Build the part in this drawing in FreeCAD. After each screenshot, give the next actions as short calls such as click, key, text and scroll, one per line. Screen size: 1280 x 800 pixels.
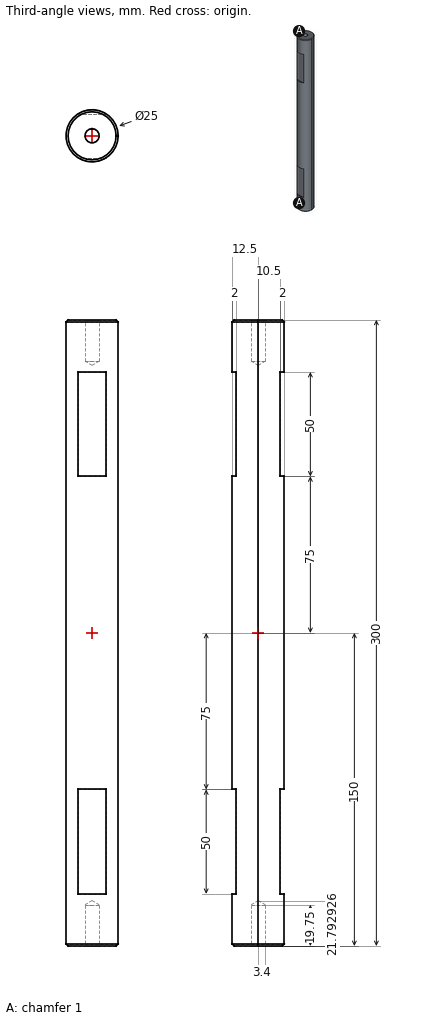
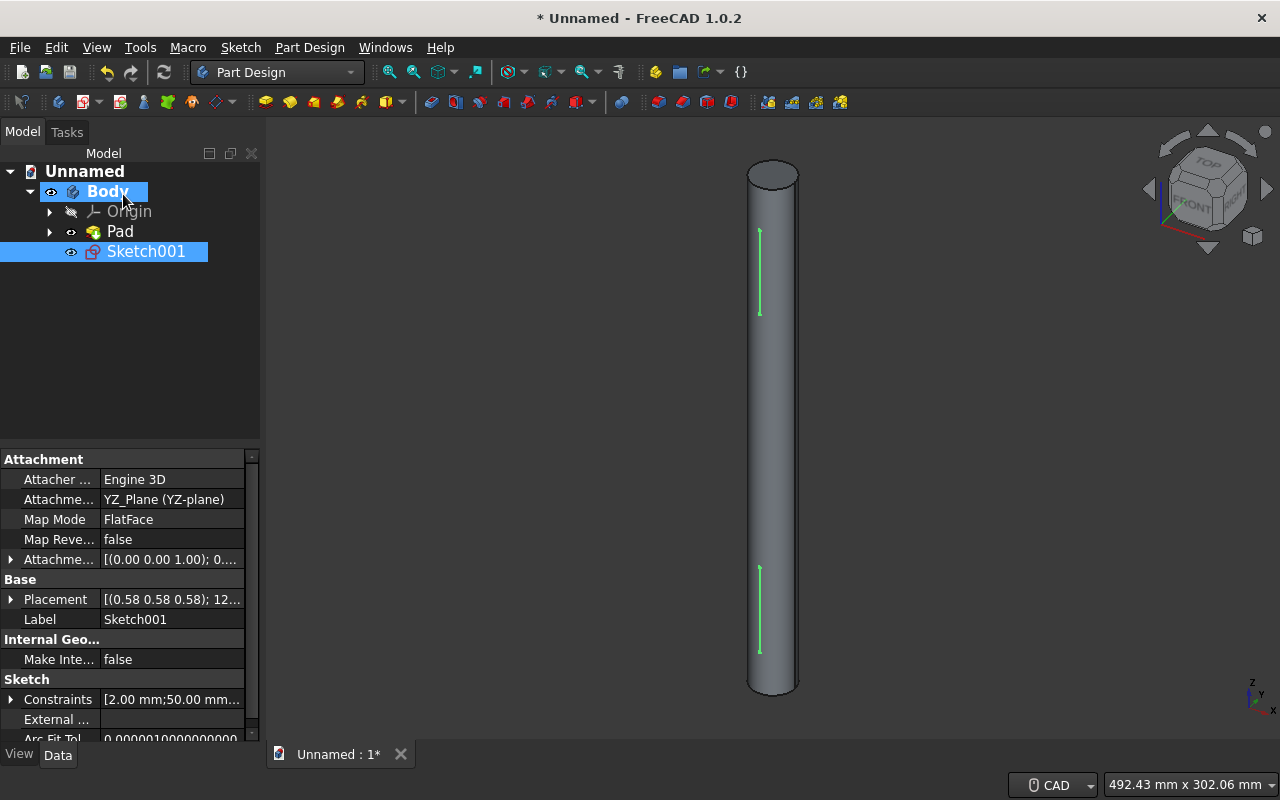
click(432, 102)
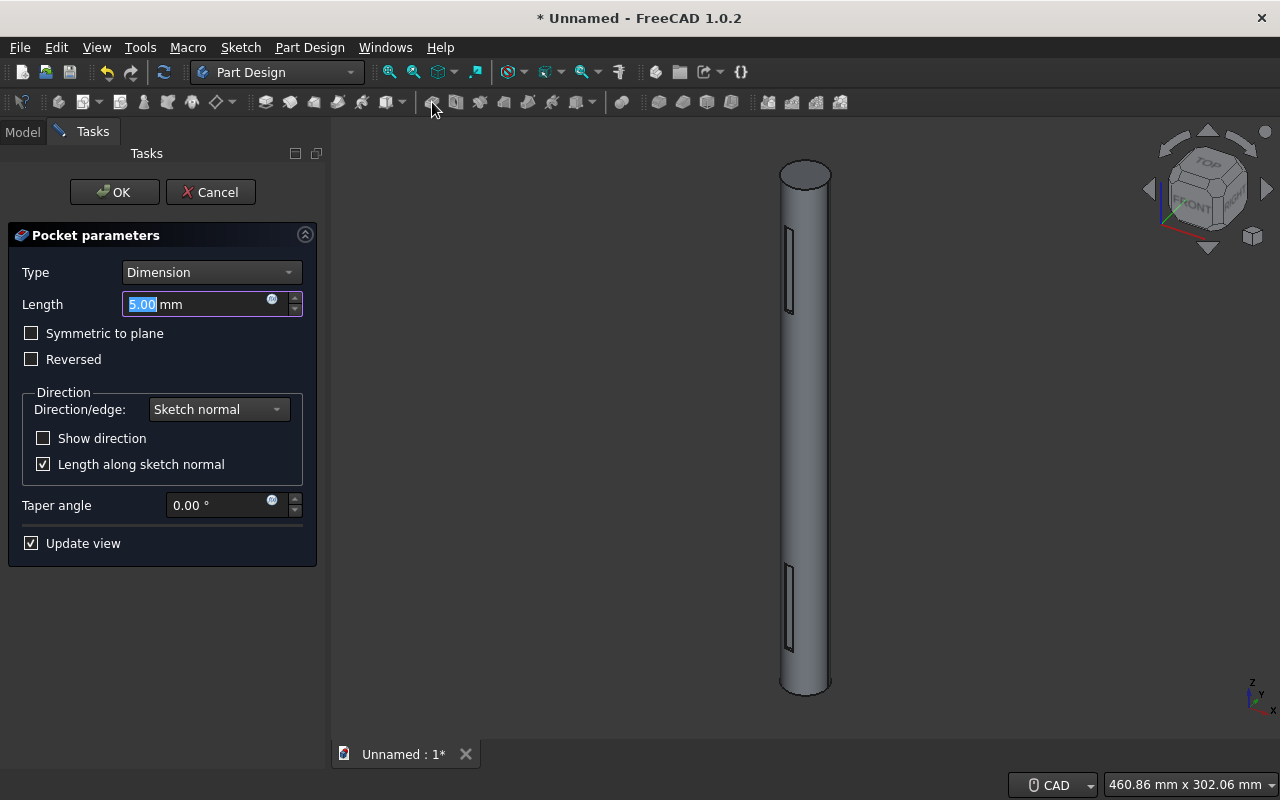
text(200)
key(Tab)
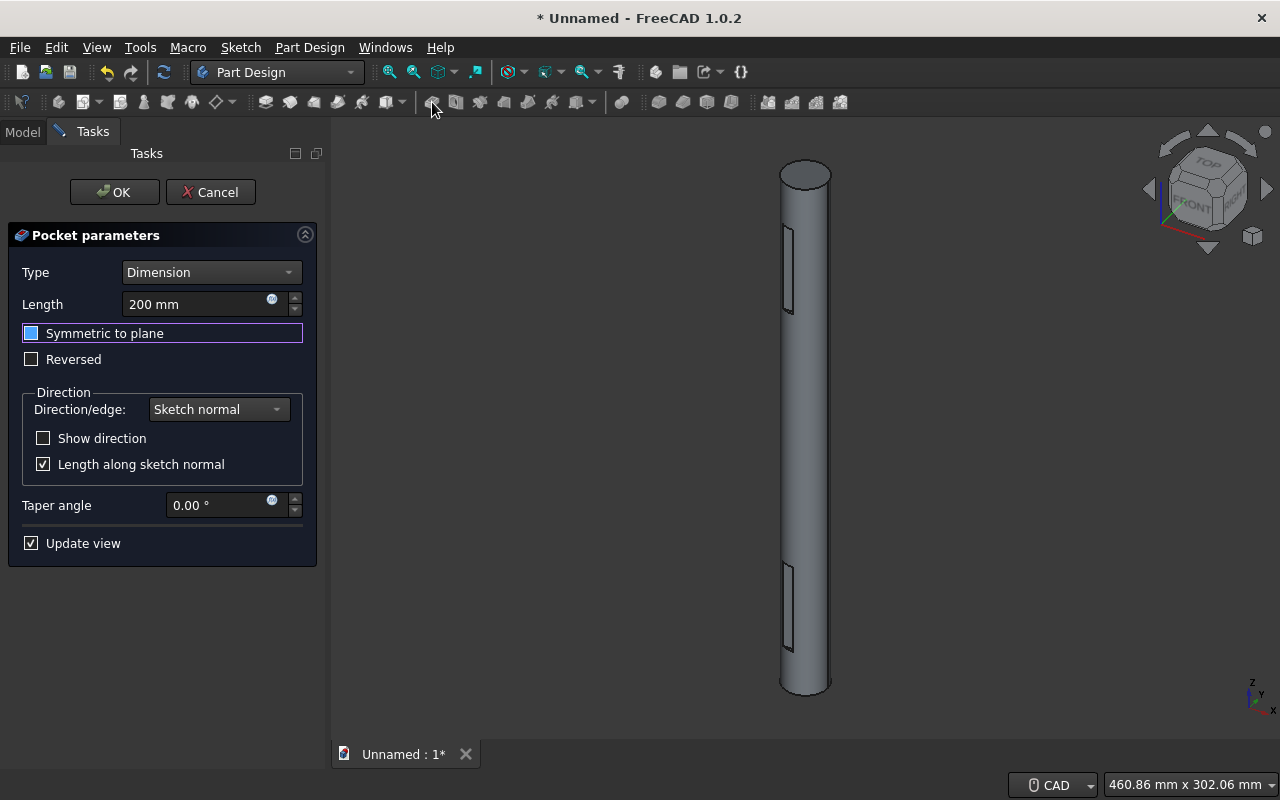
click(30, 333)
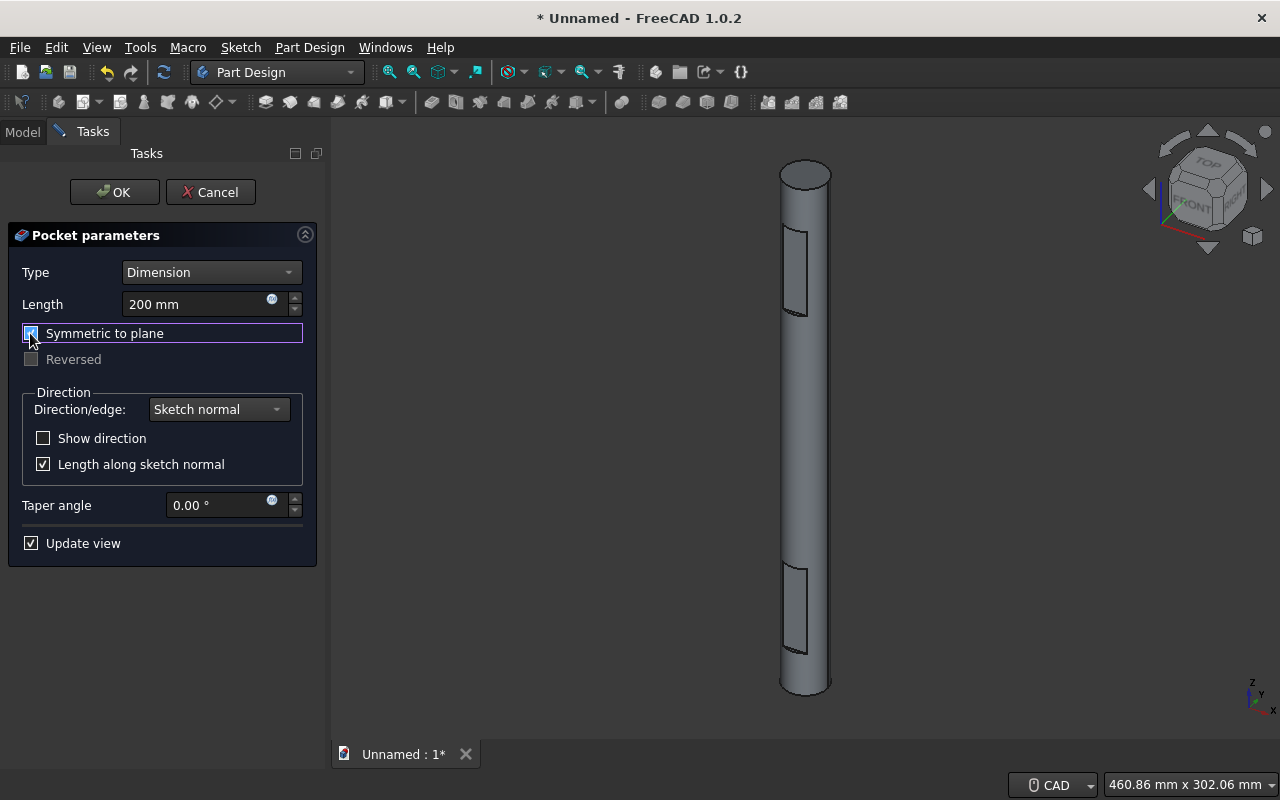
click(115, 192)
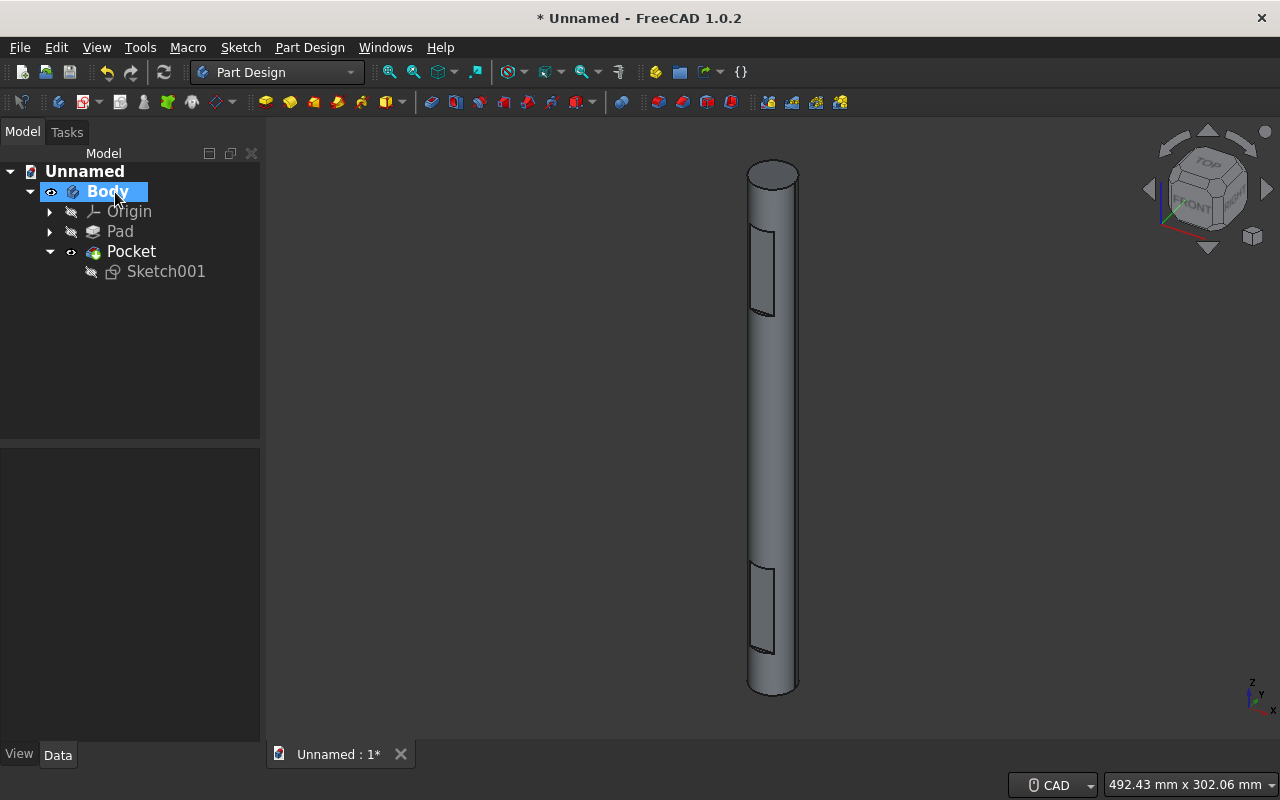
click(747, 176)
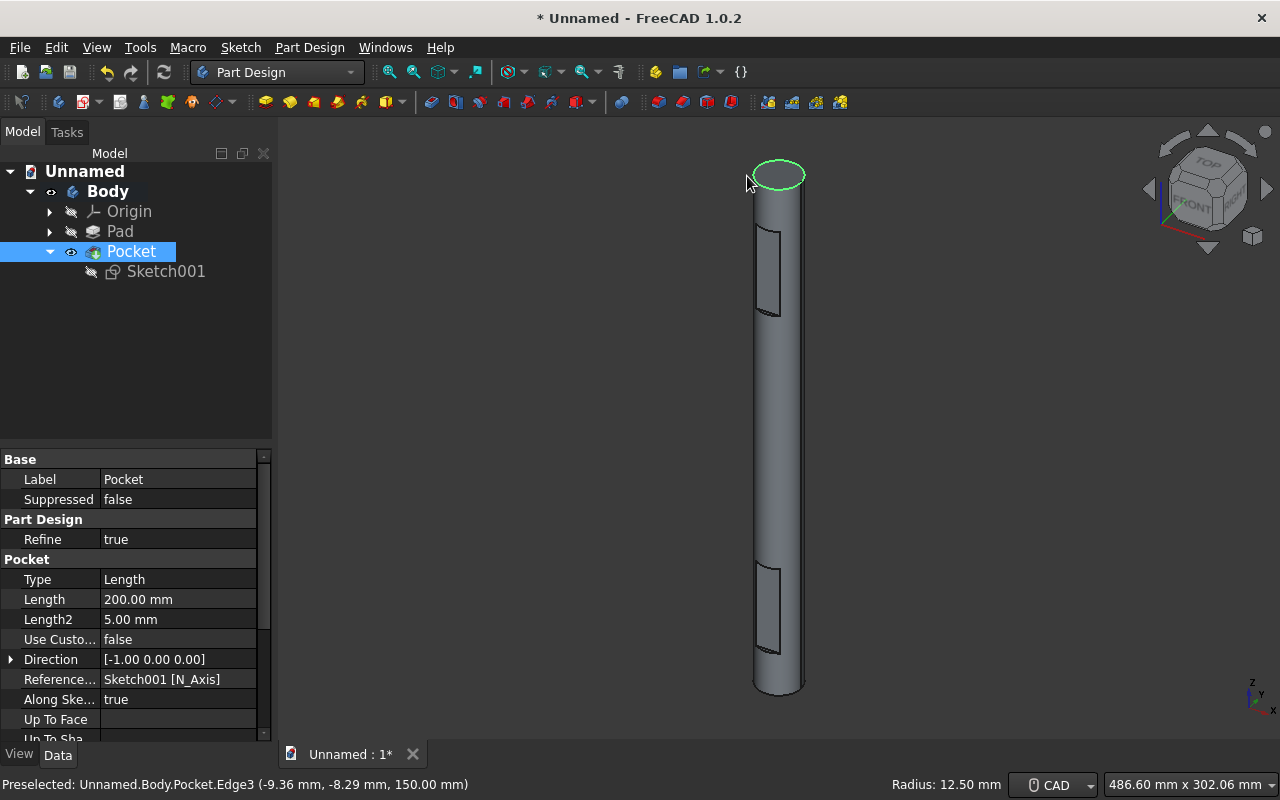
key(0)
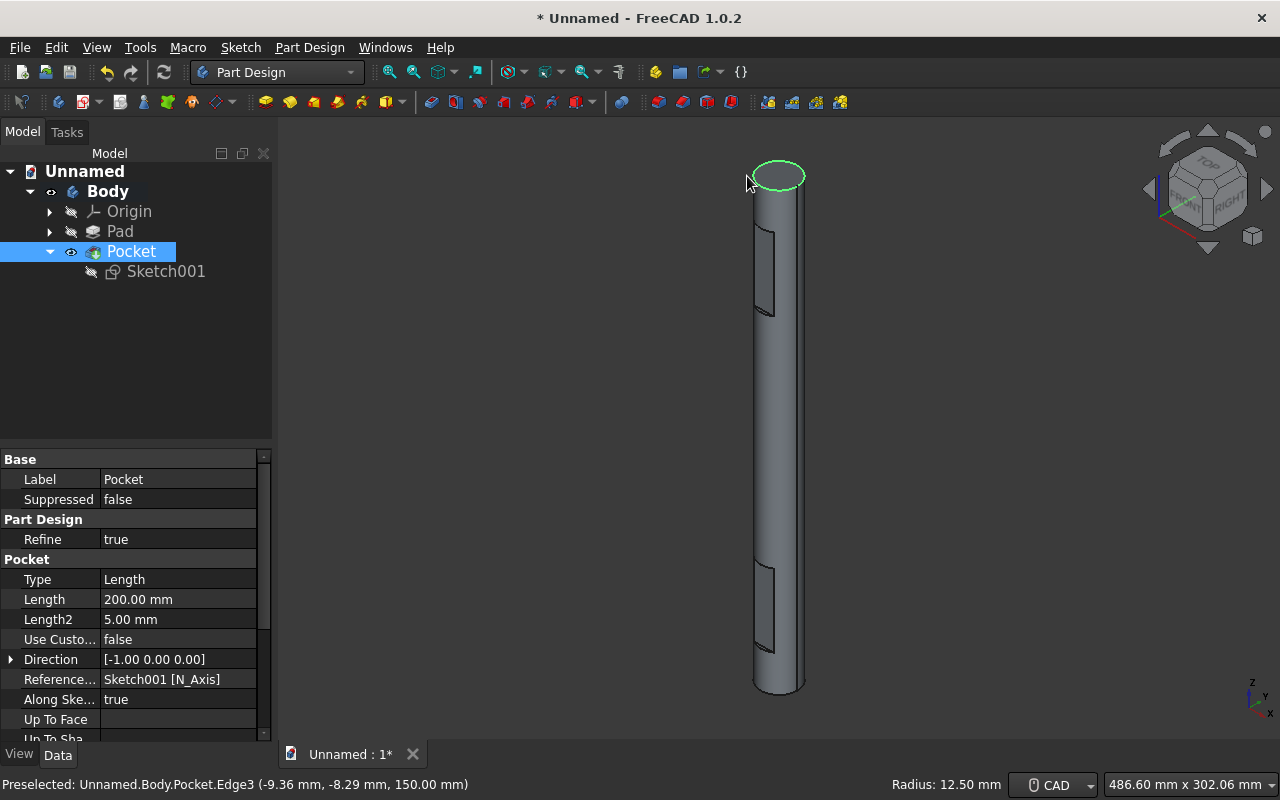
click(756, 686, ctrl)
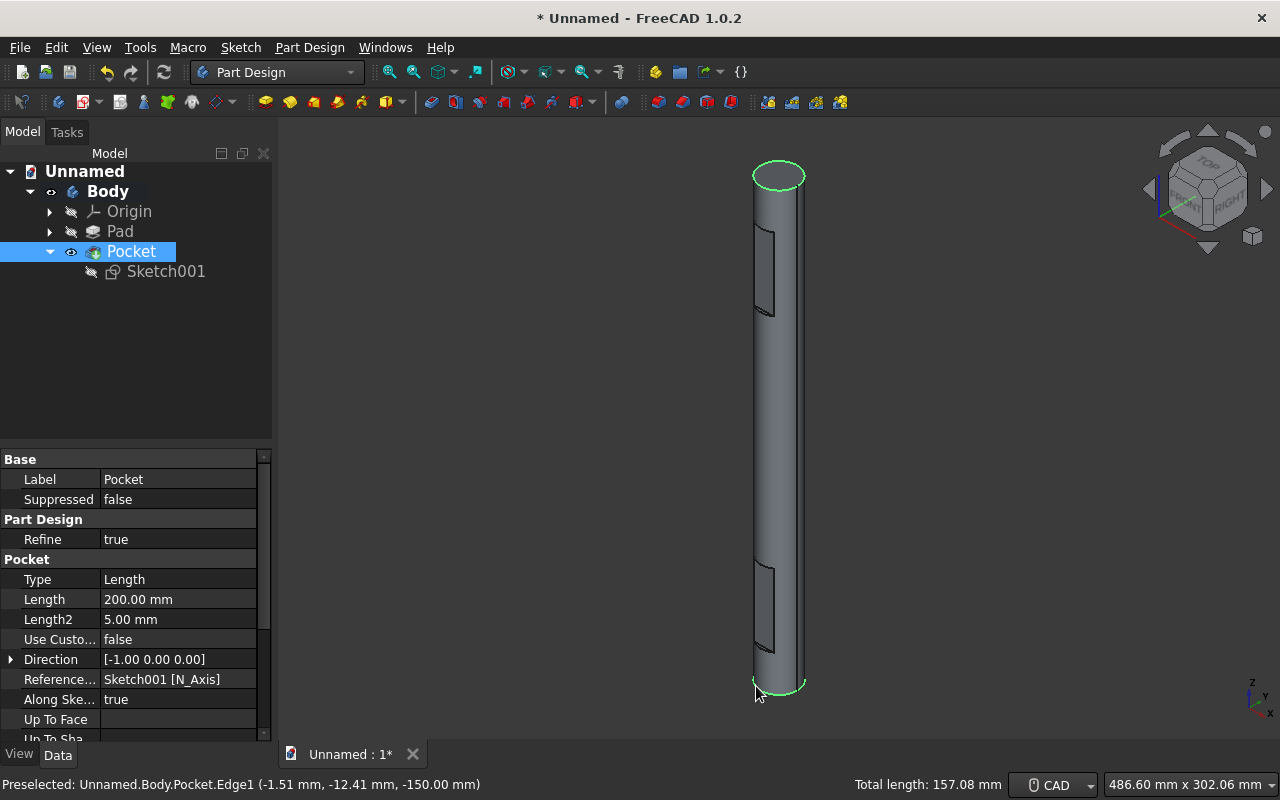
click(684, 102)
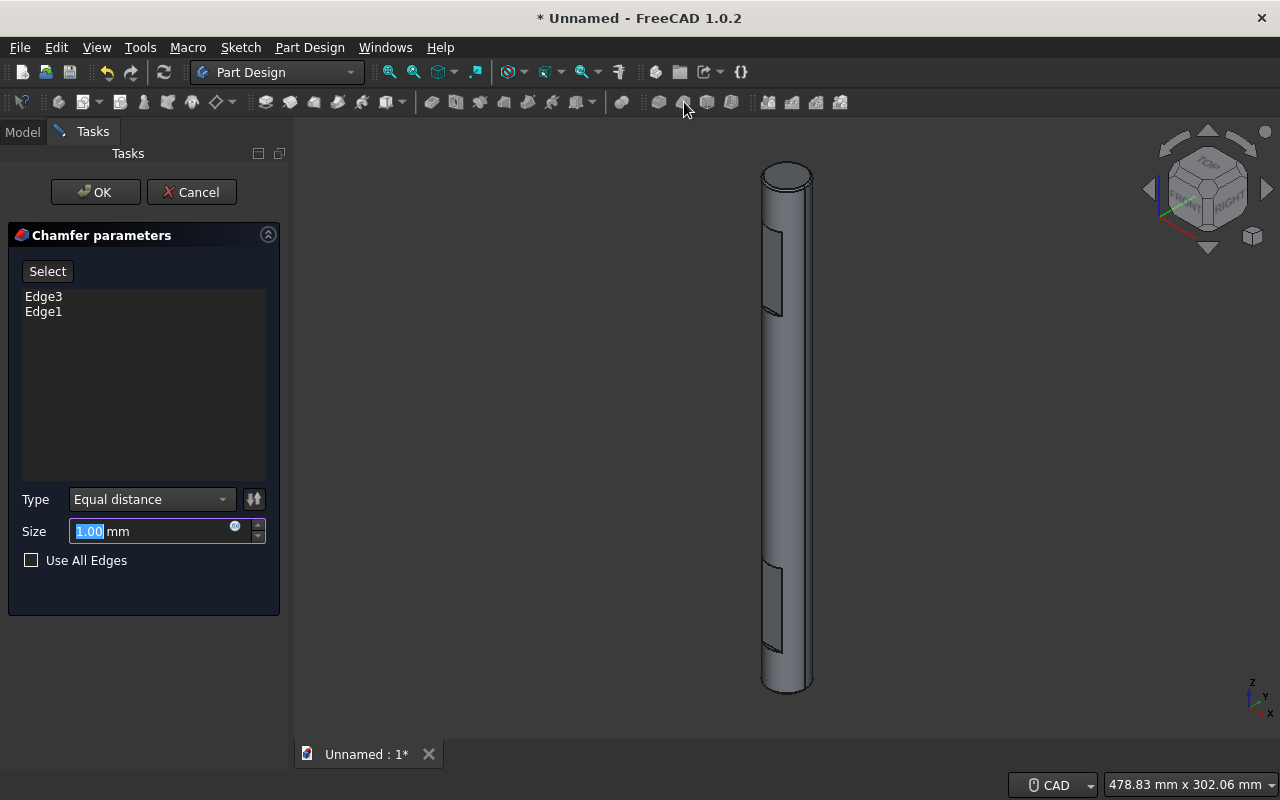
text(1)
key(Tab)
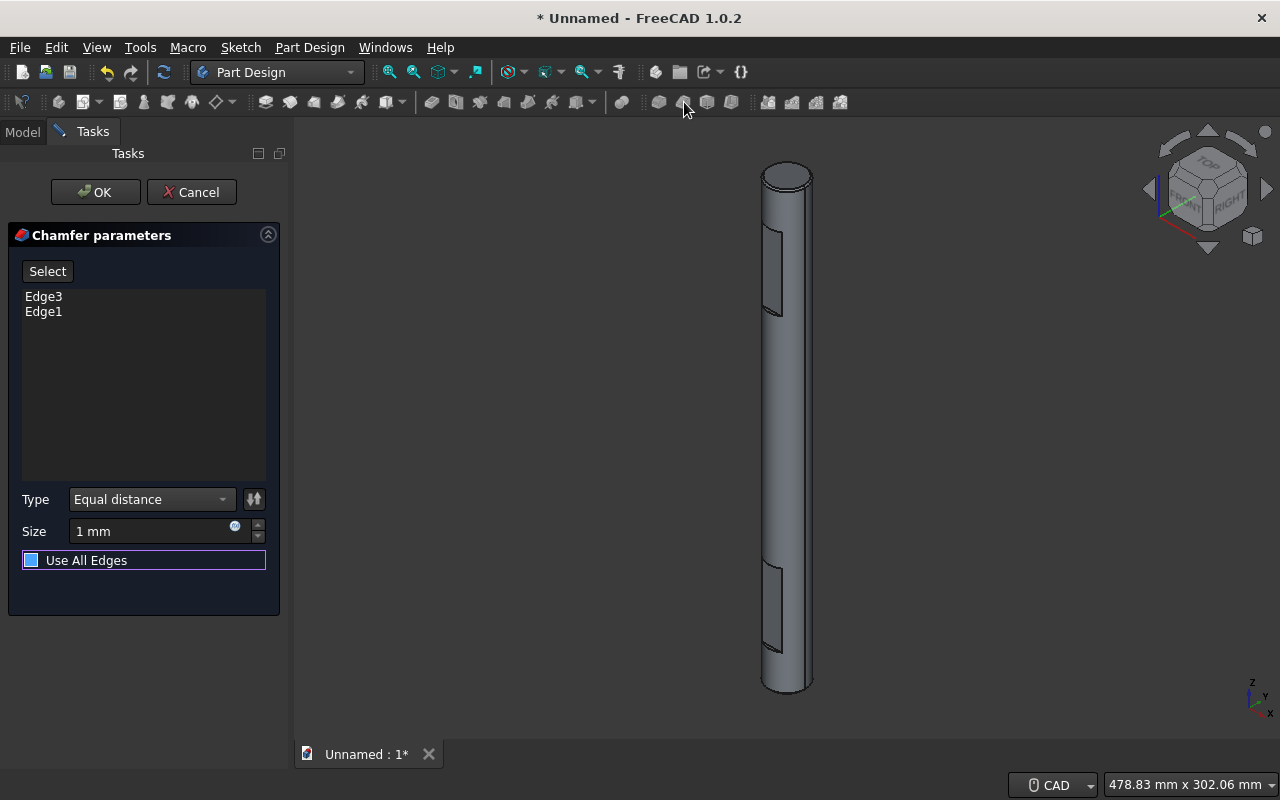
click(96, 192)